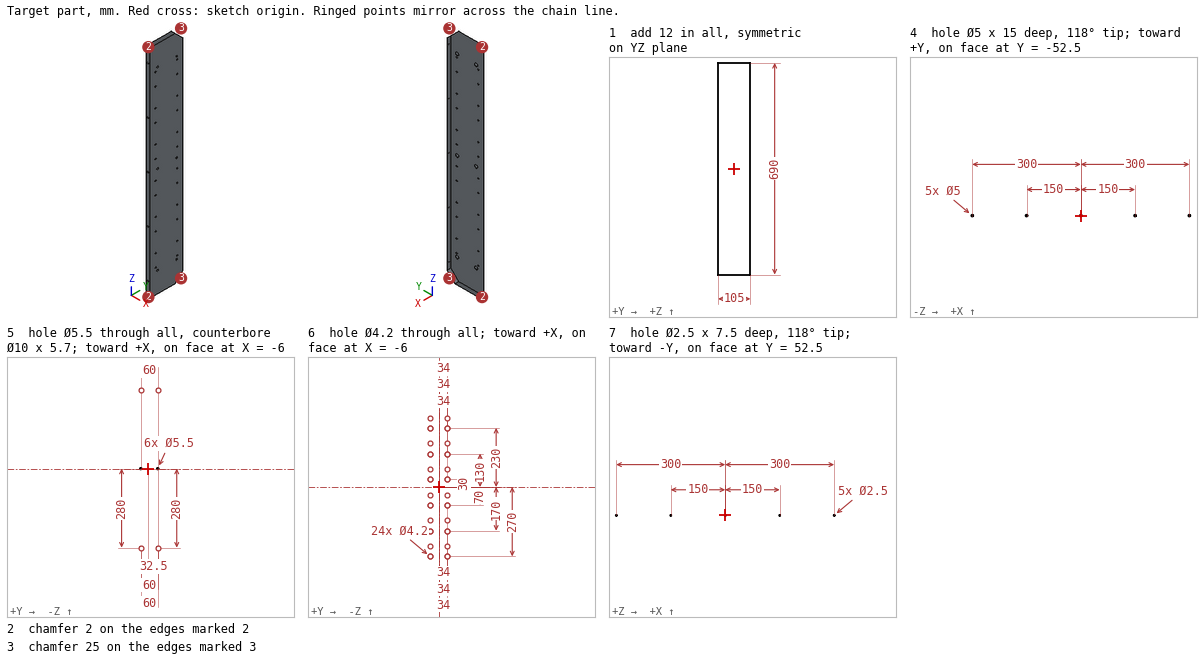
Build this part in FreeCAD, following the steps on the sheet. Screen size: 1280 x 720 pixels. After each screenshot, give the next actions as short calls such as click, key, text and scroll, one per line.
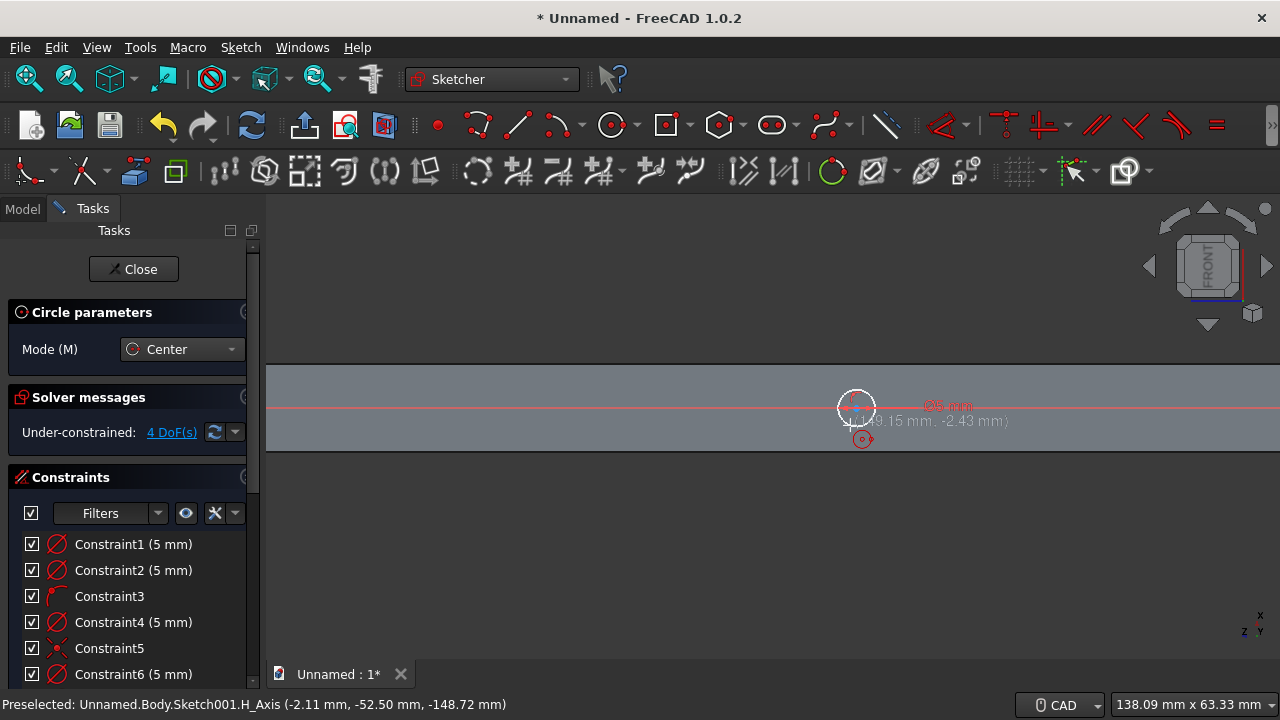
scroll(853, 429, down, 10)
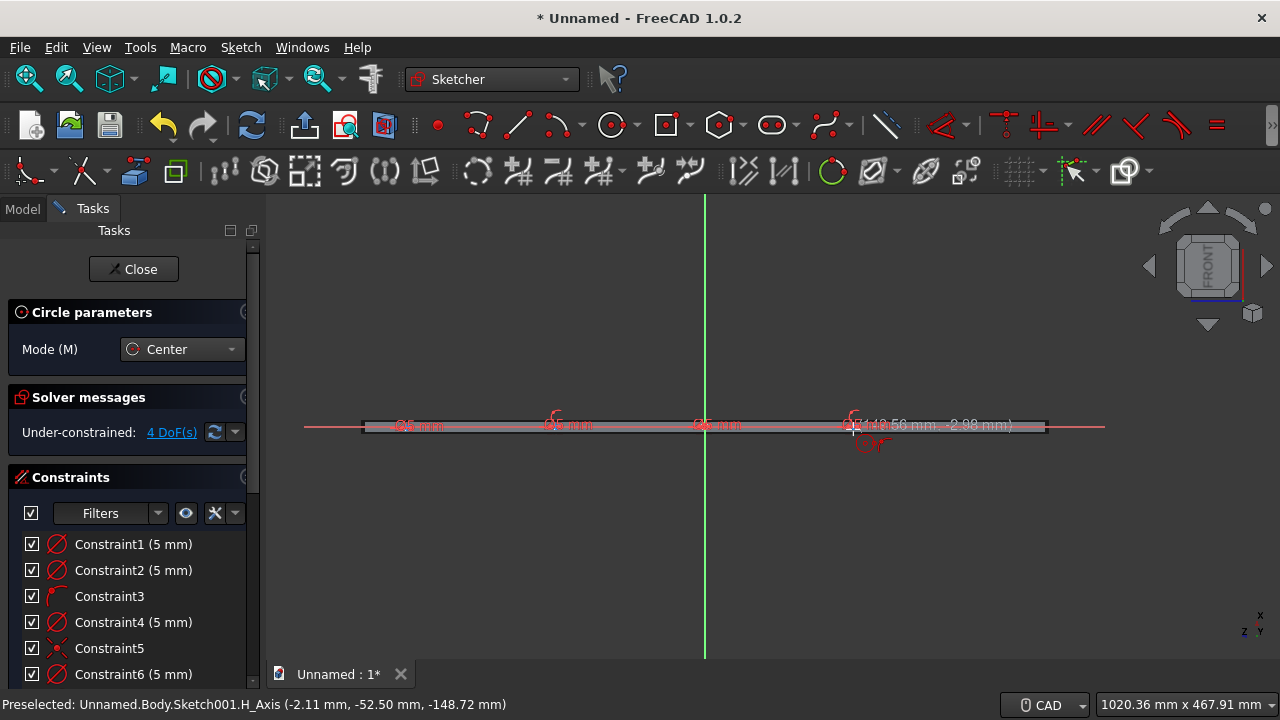
scroll(1003, 427, up, 12)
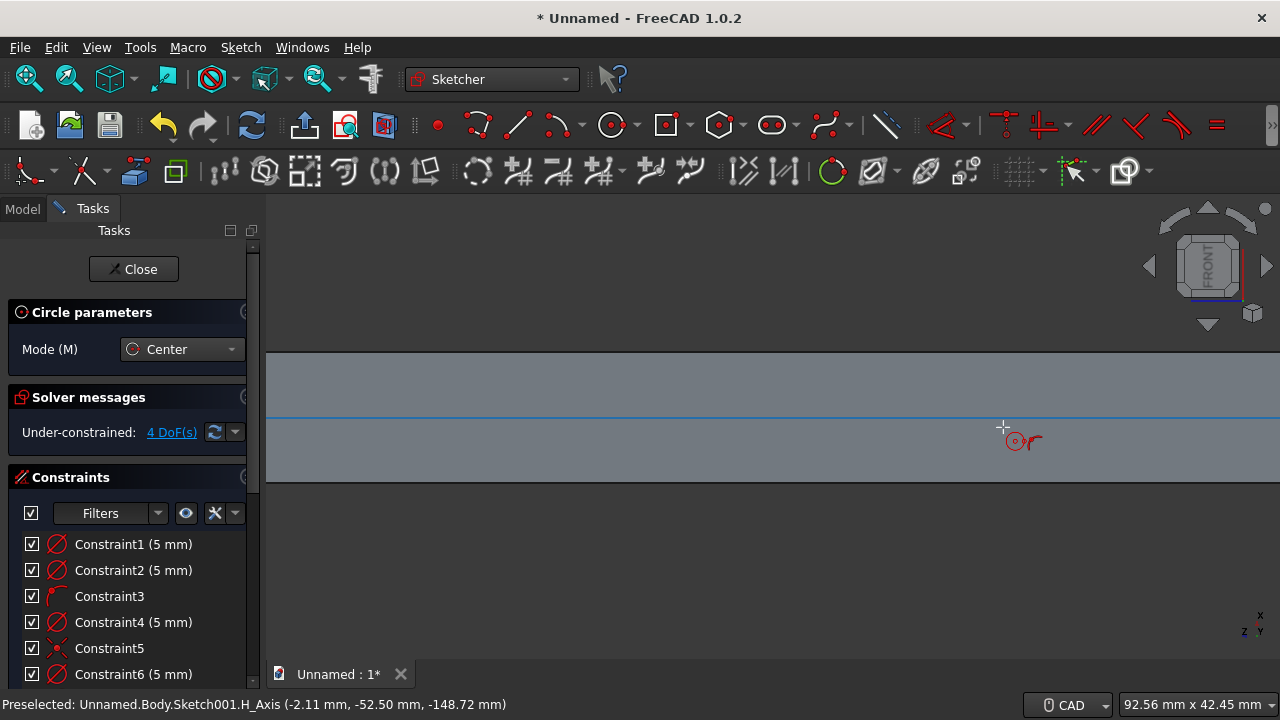
scroll(1003, 427, down, 12)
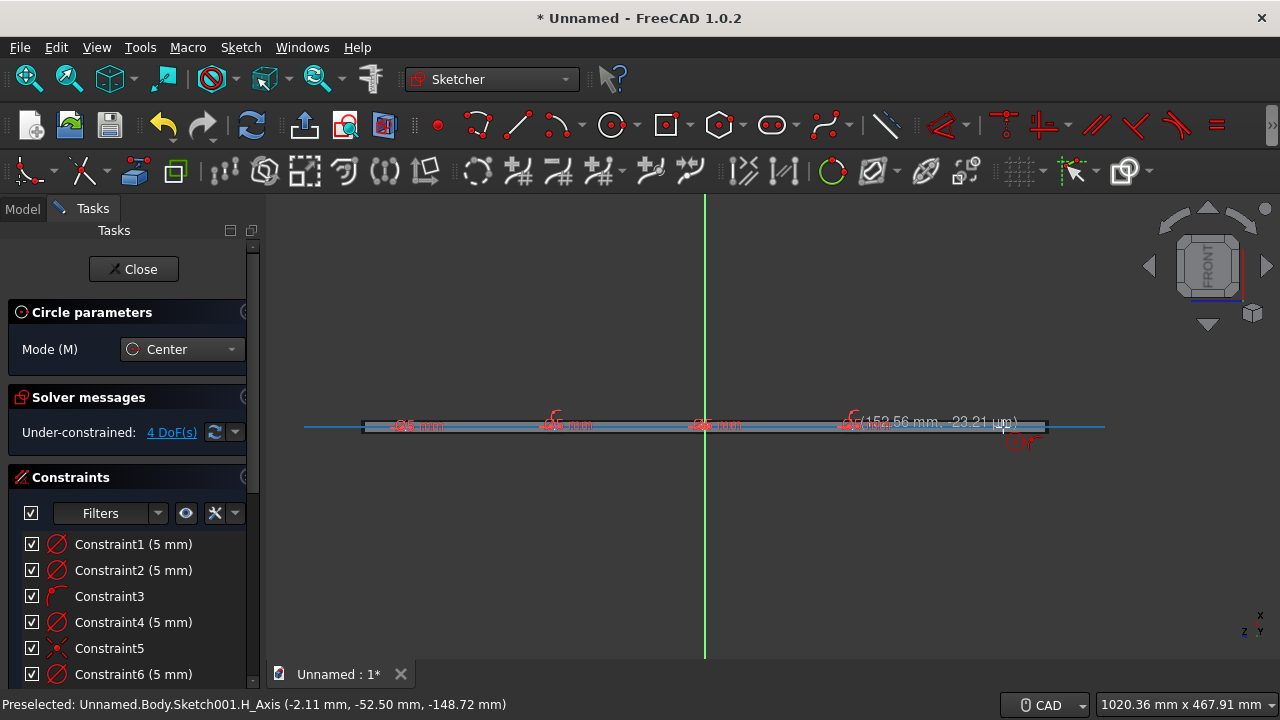
click(1003, 427)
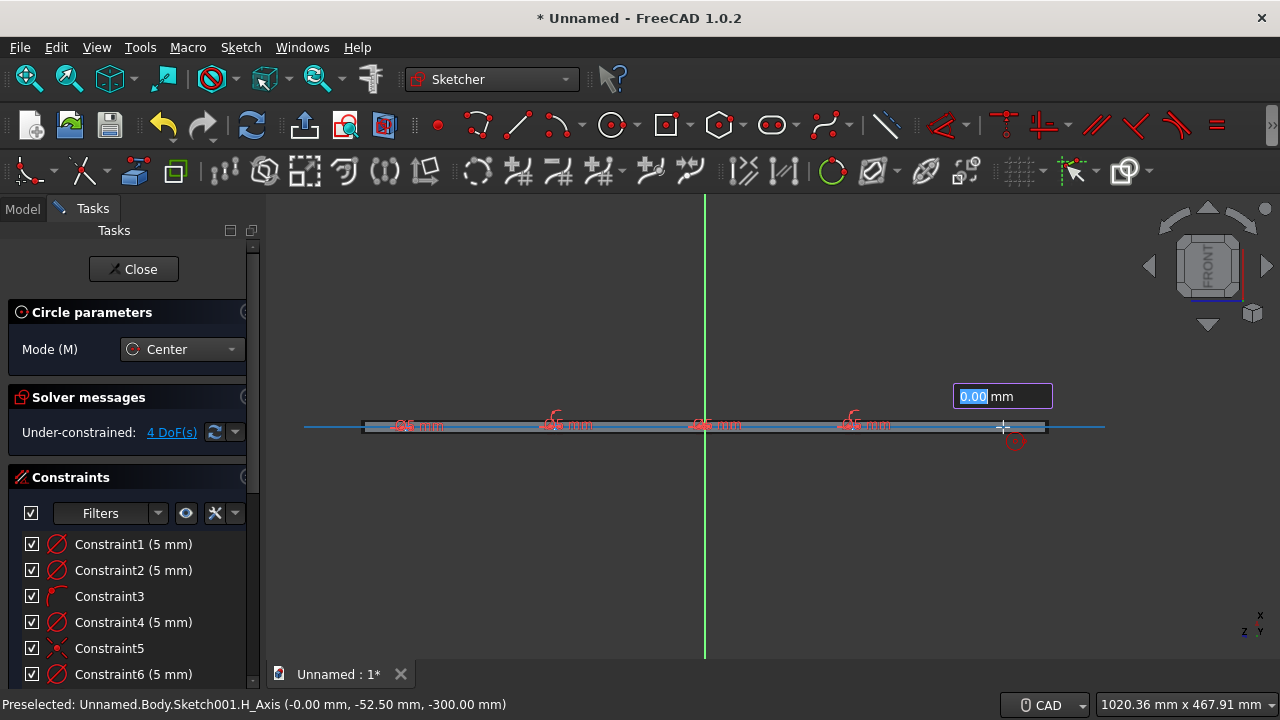
scroll(1002, 429, up, 10)
move(998, 425)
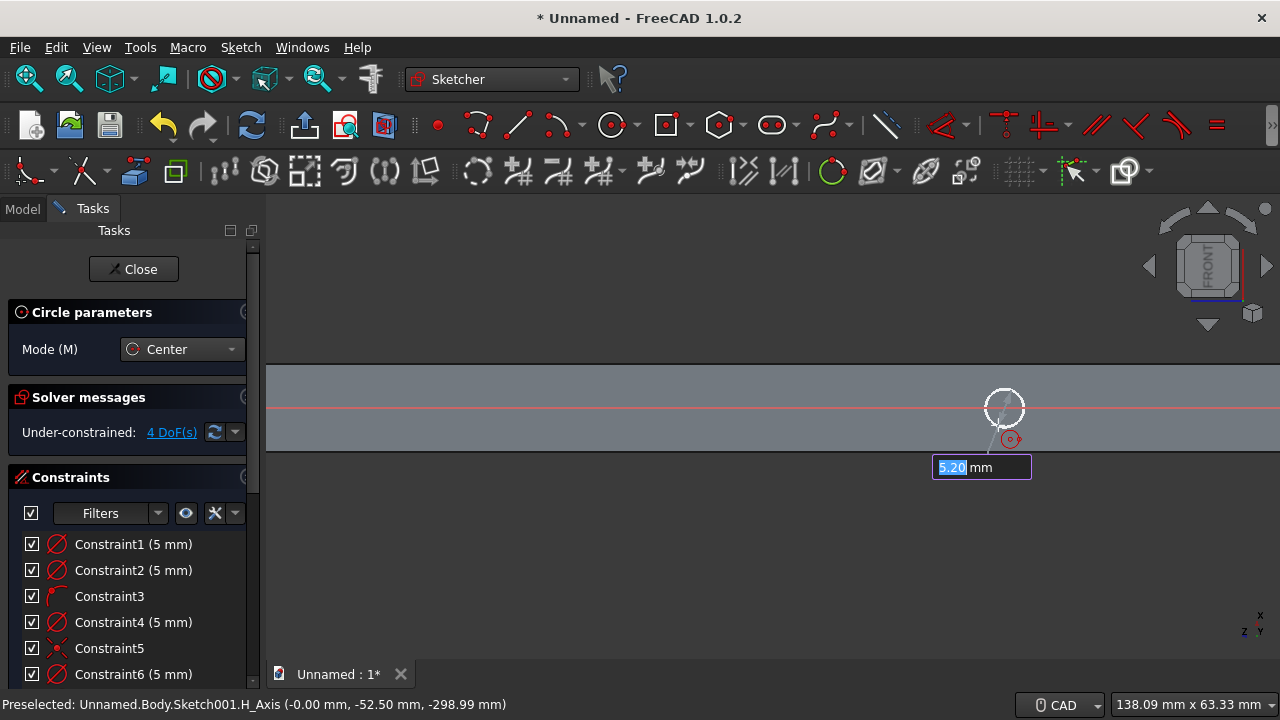
text(5)
key(Return)
key(Escape)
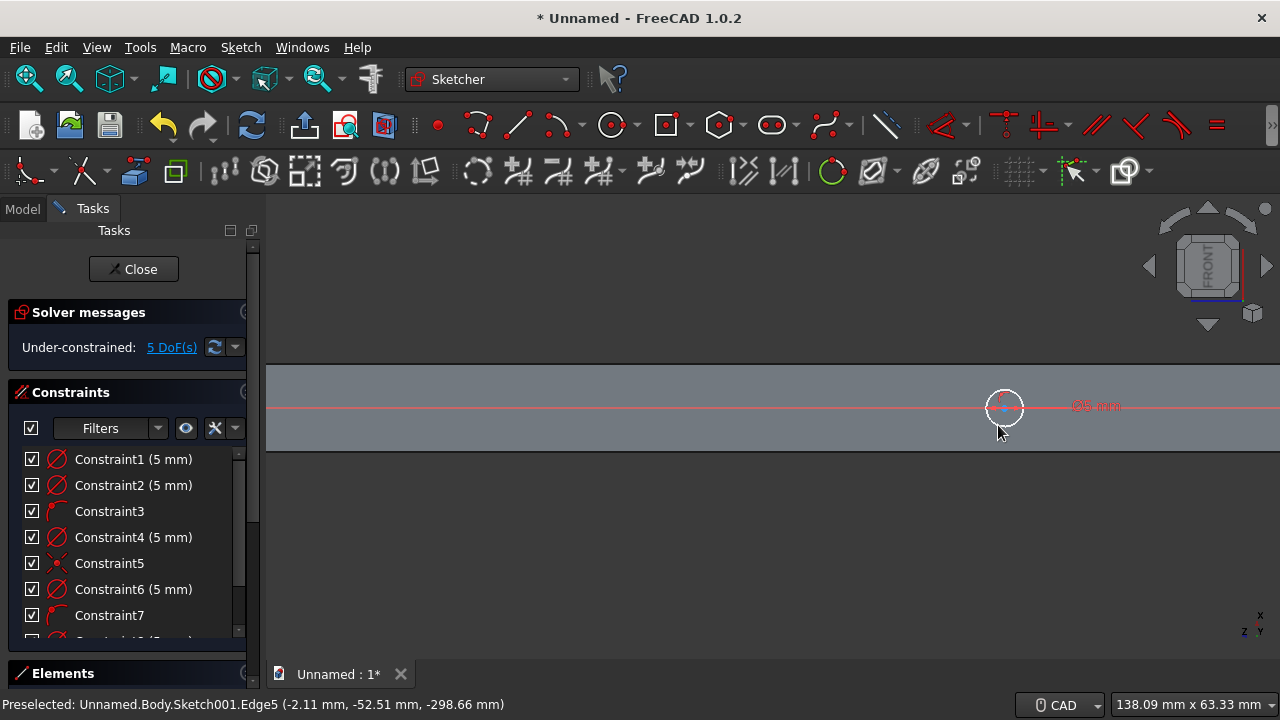
scroll(1002, 429, down, 10)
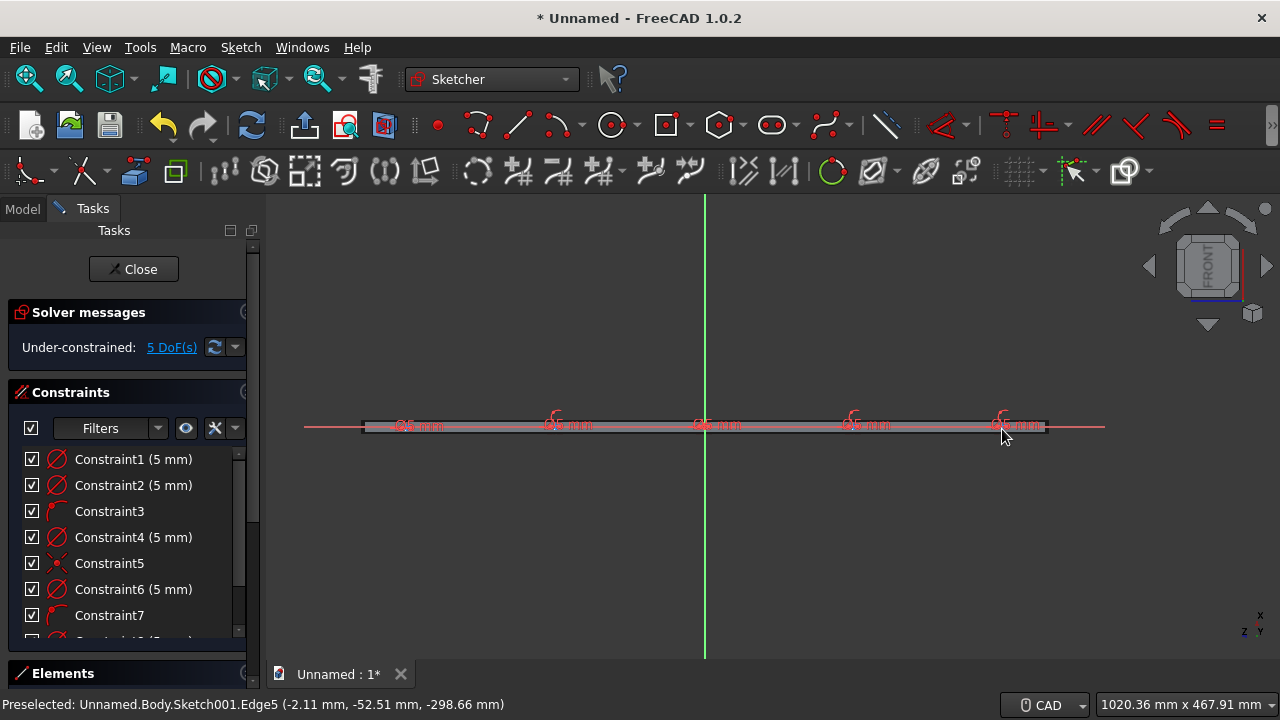
click(407, 428)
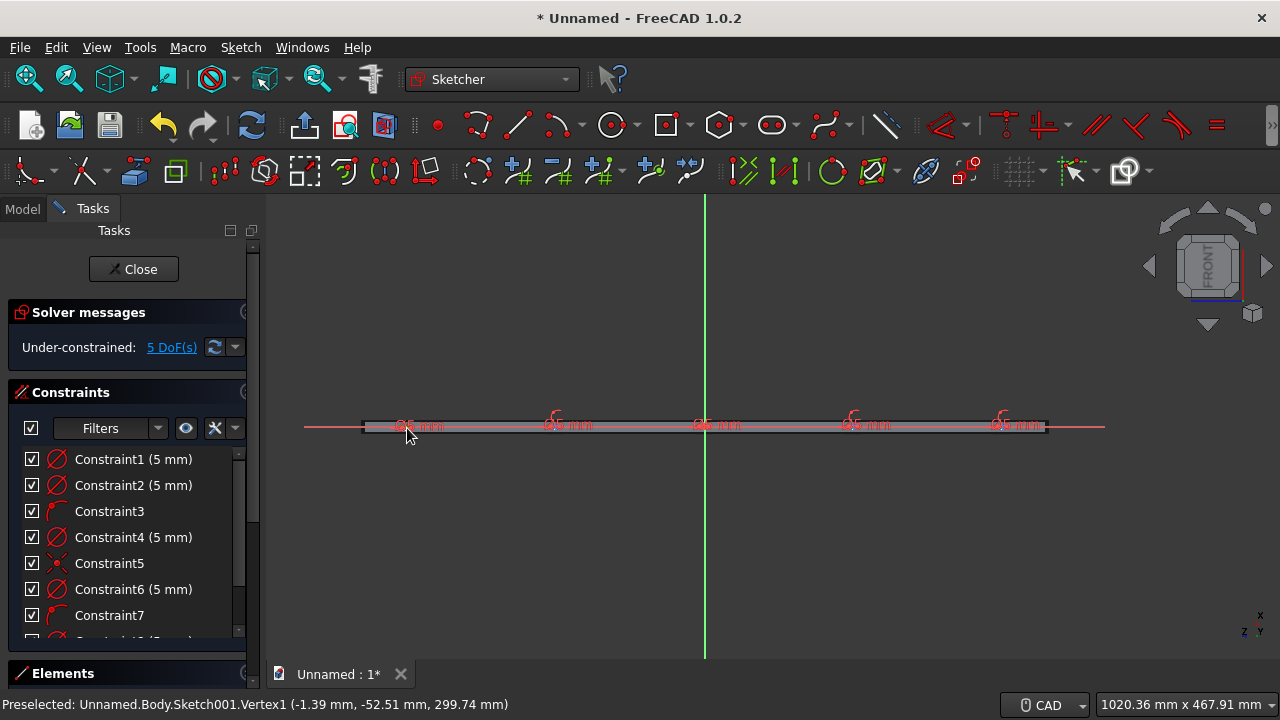
click(353, 427)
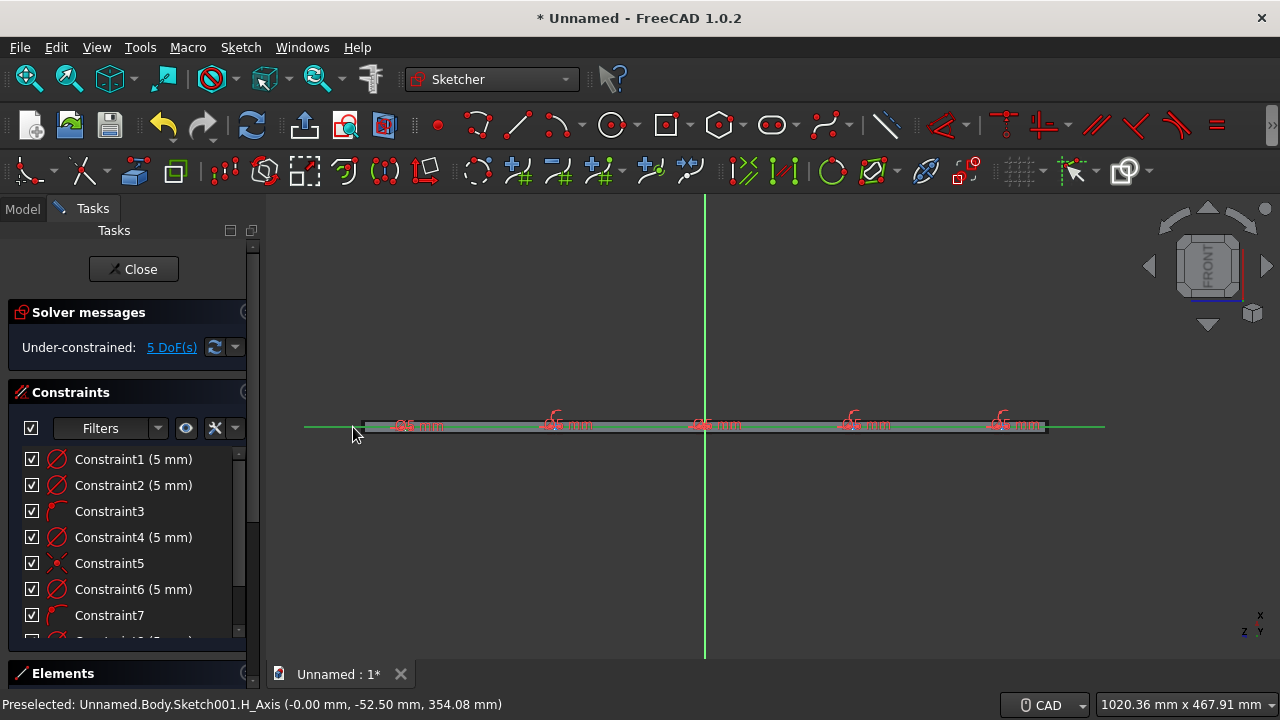
click(1004, 126)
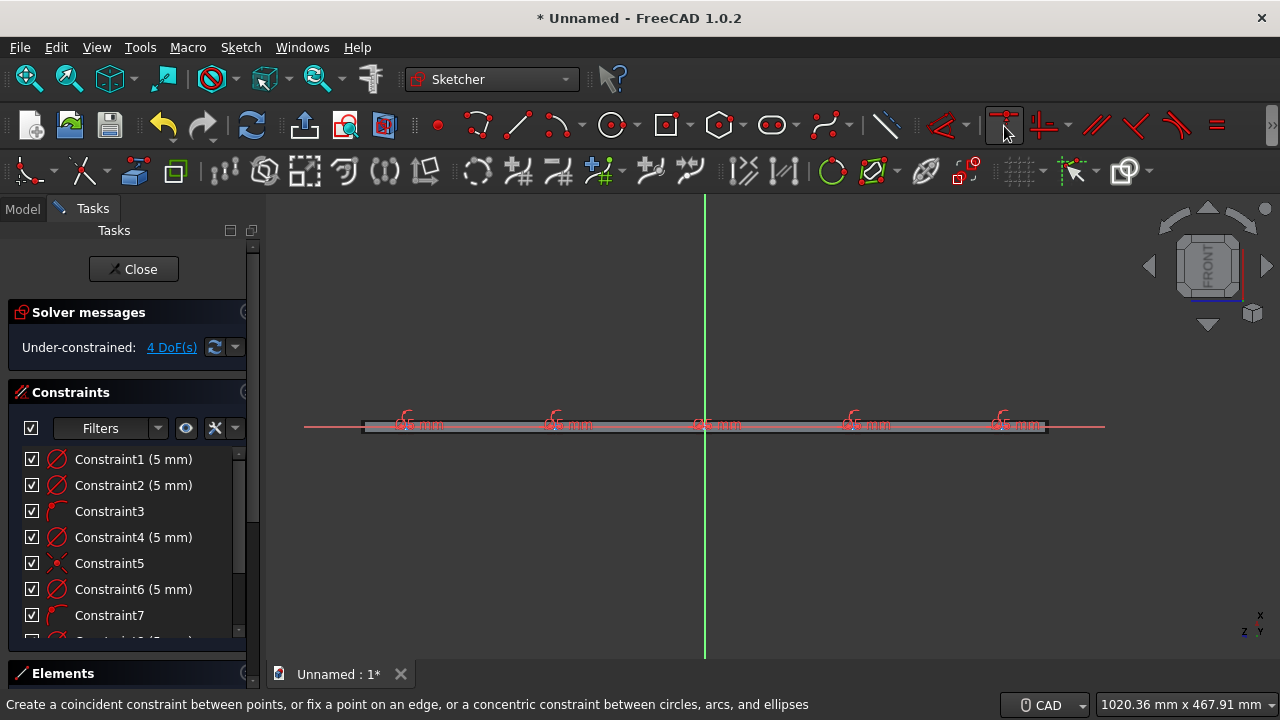
click(942, 126)